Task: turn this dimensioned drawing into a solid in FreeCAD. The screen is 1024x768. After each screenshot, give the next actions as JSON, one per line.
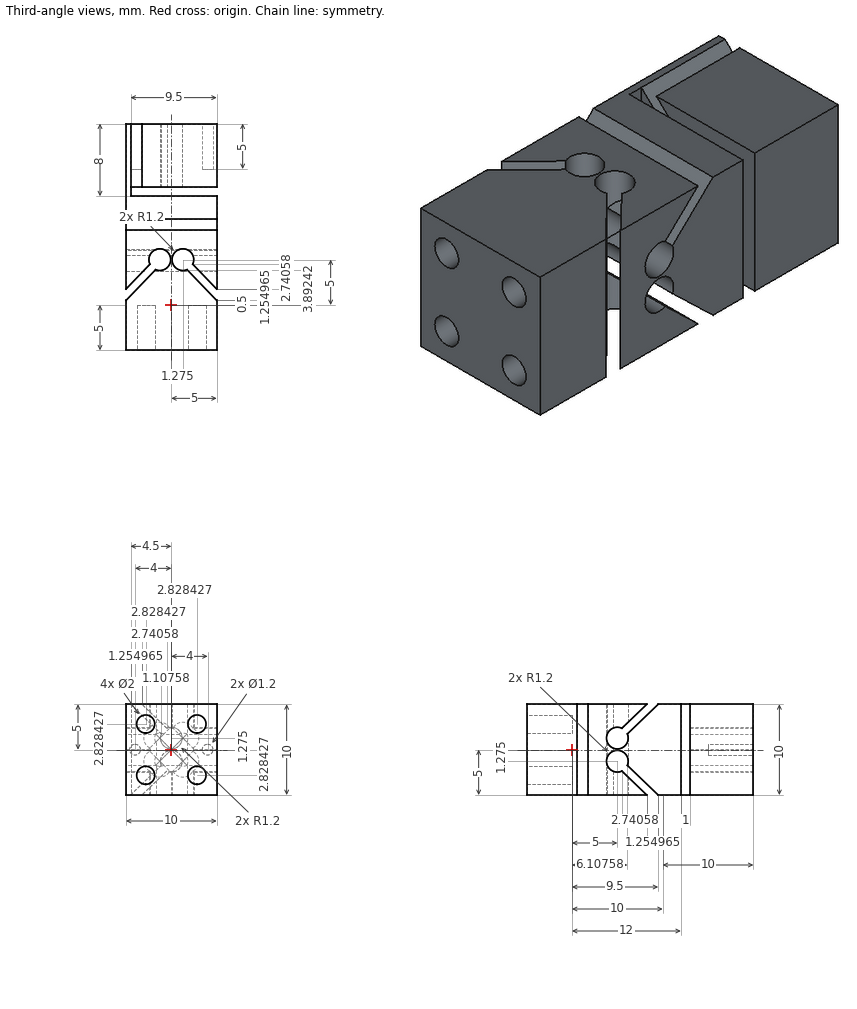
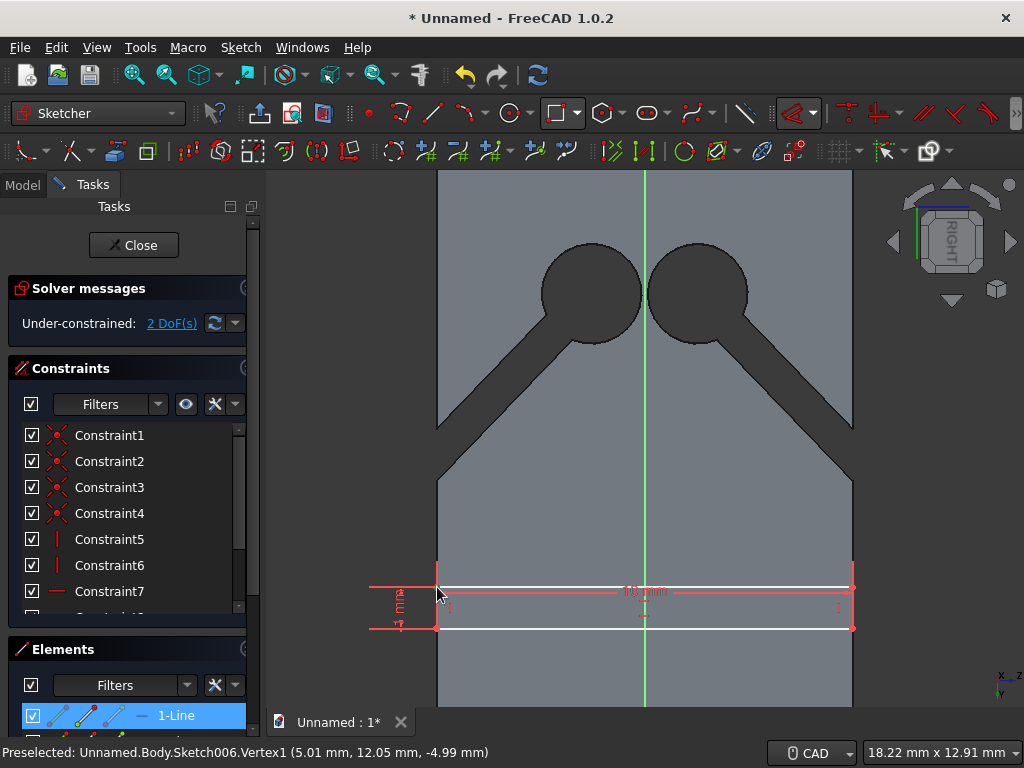
{"action": "key", "text": "l"}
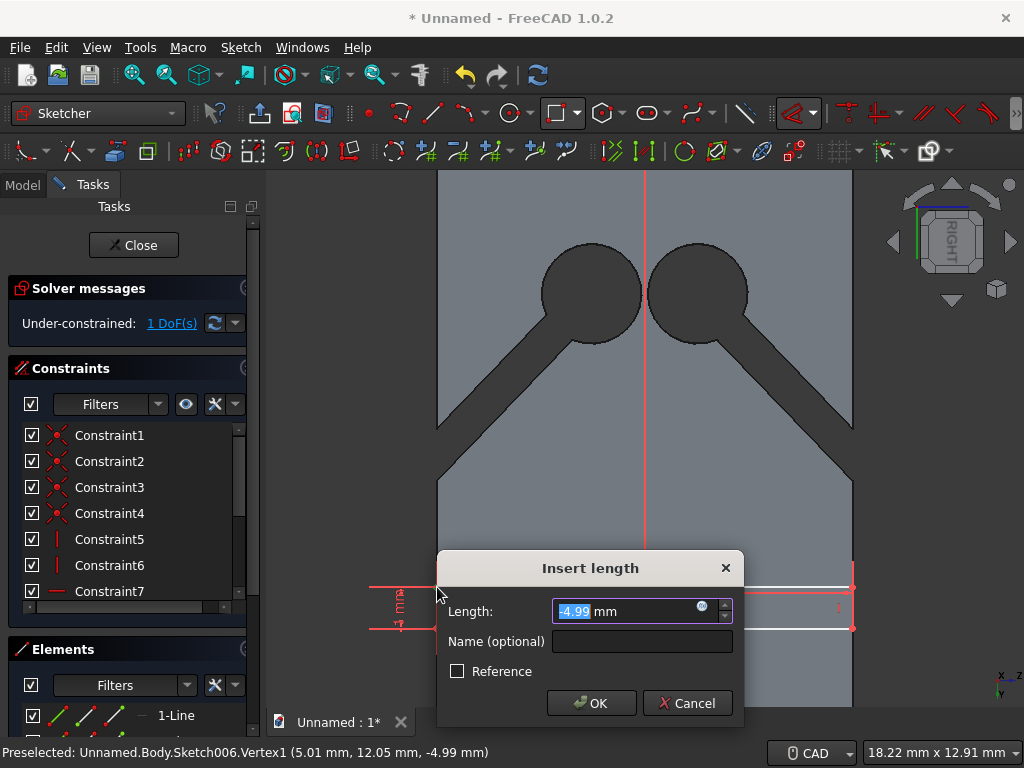
{"action": "type", "text": "-5"}
{"action": "key", "text": "Return"}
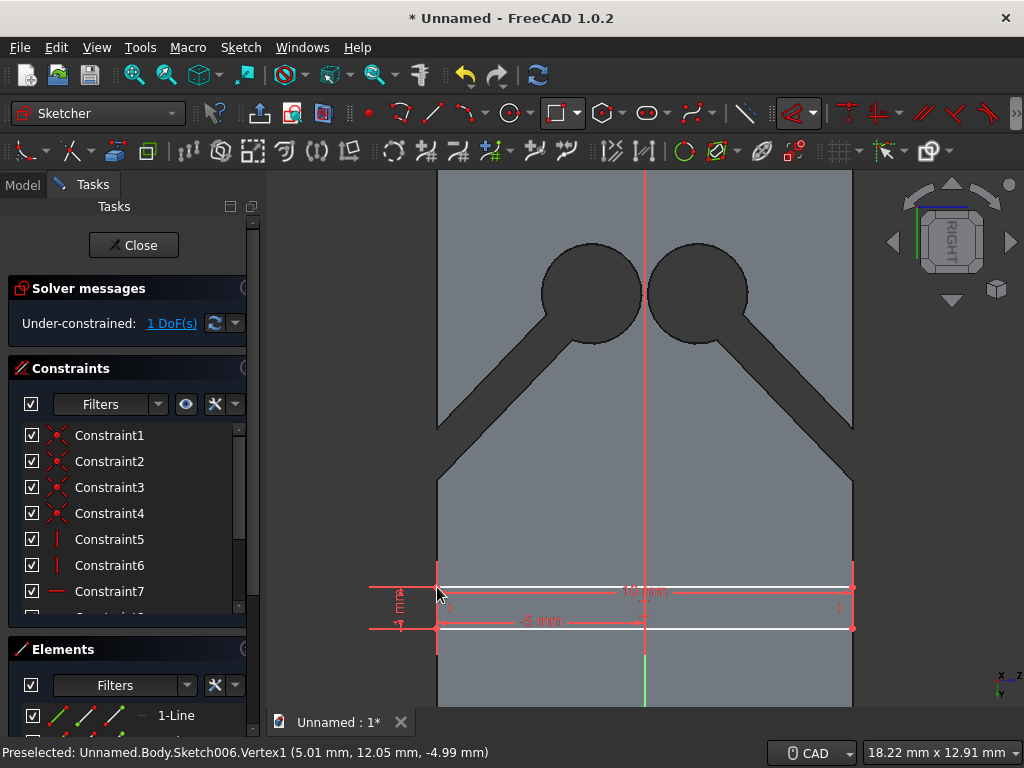
{"action": "left_click", "coordinate": [437, 587]}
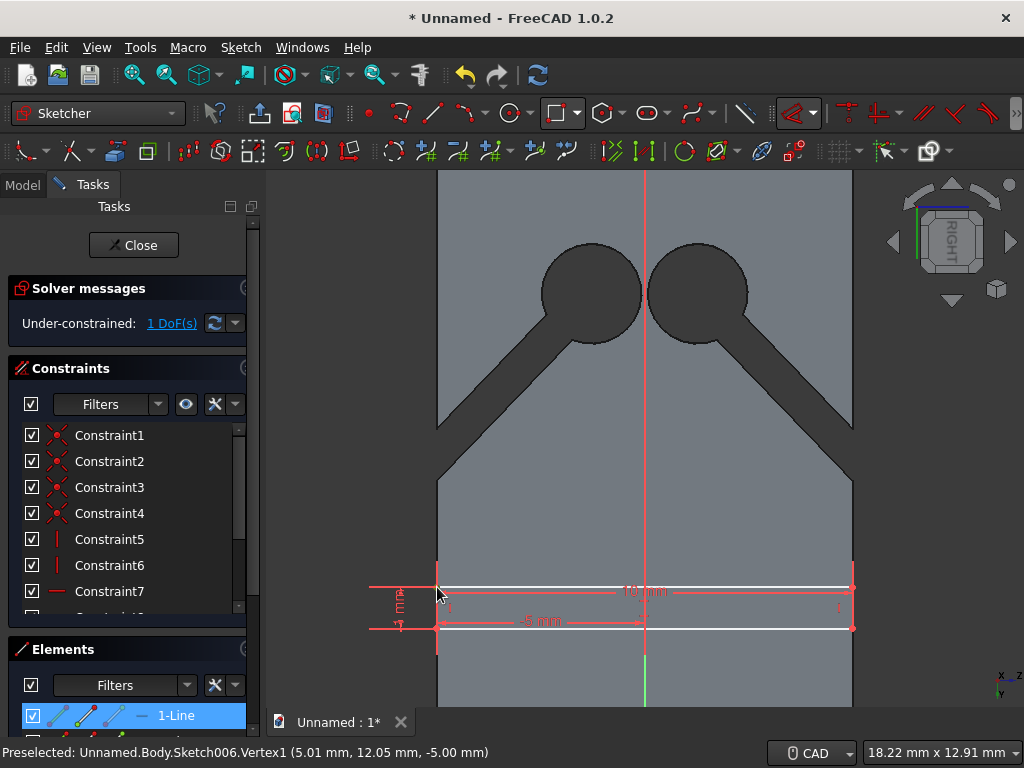
{"action": "key", "text": "i"}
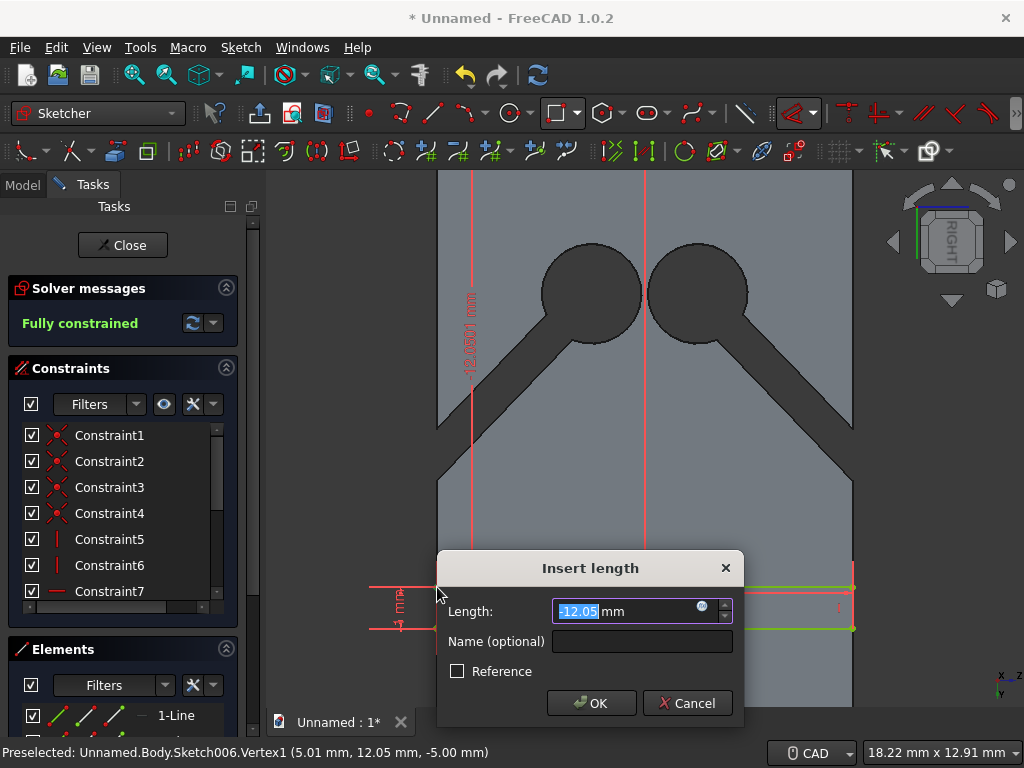
{"action": "type", "text": "-12"}
{"action": "key", "text": "Return"}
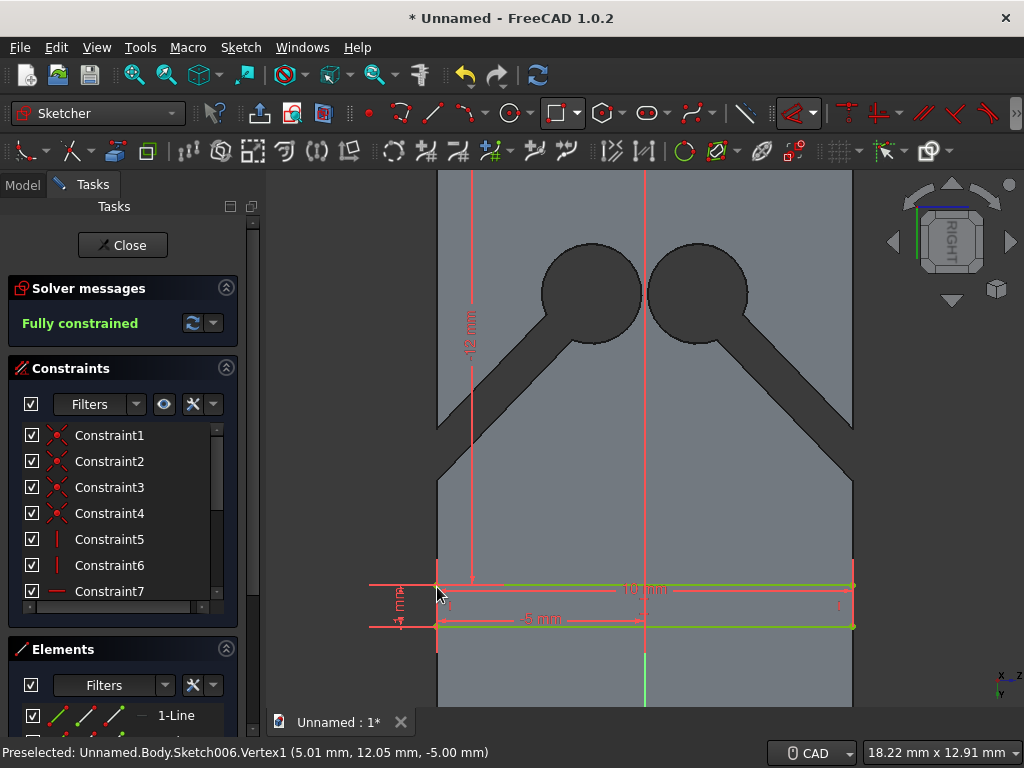
{"action": "left_click", "coordinate": [123, 245]}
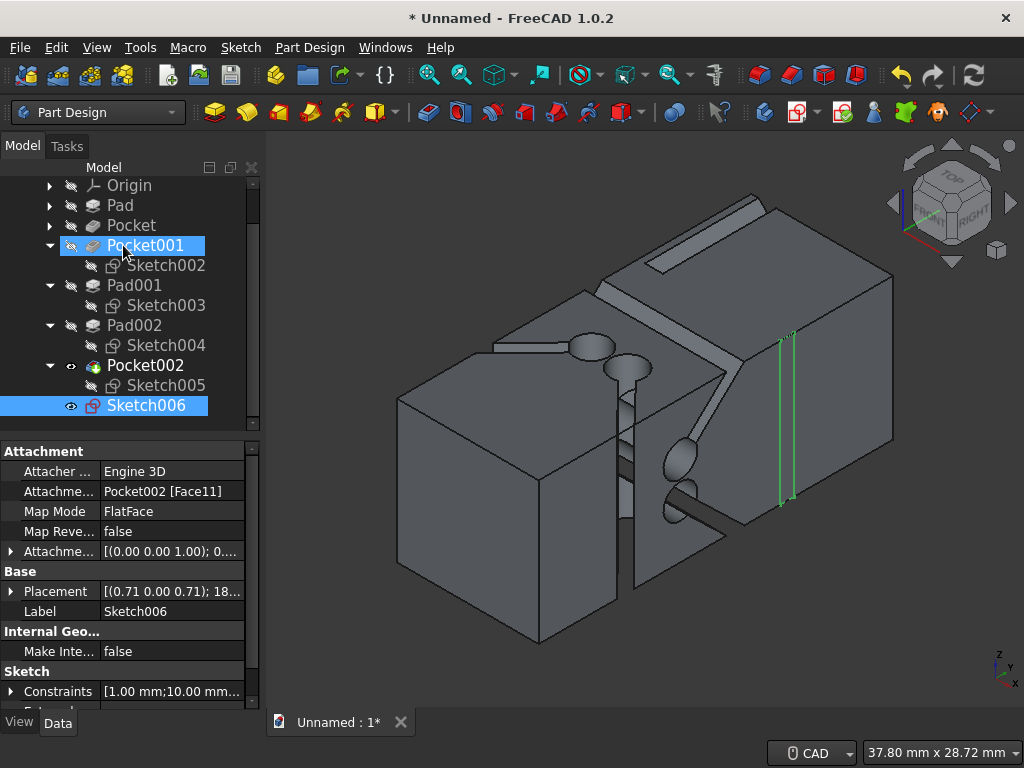
{"action": "left_click", "coordinate": [430, 112]}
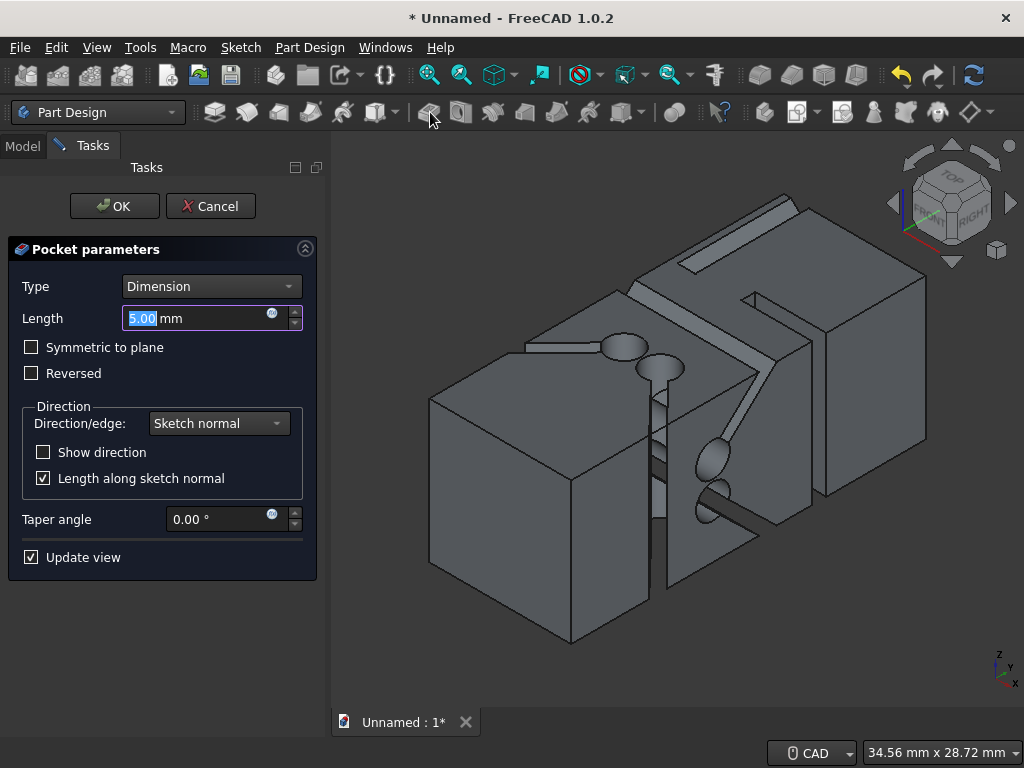
{"action": "type", "text": "9.5"}
{"action": "key", "text": "Tab"}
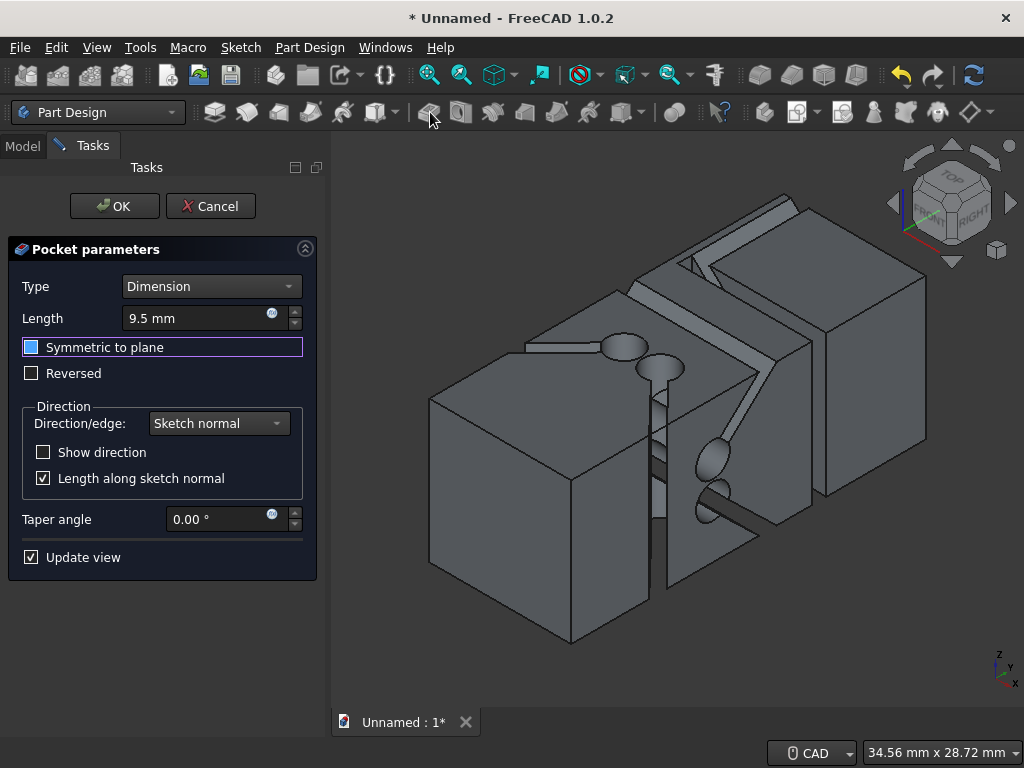
{"action": "left_click", "coordinate": [115, 206]}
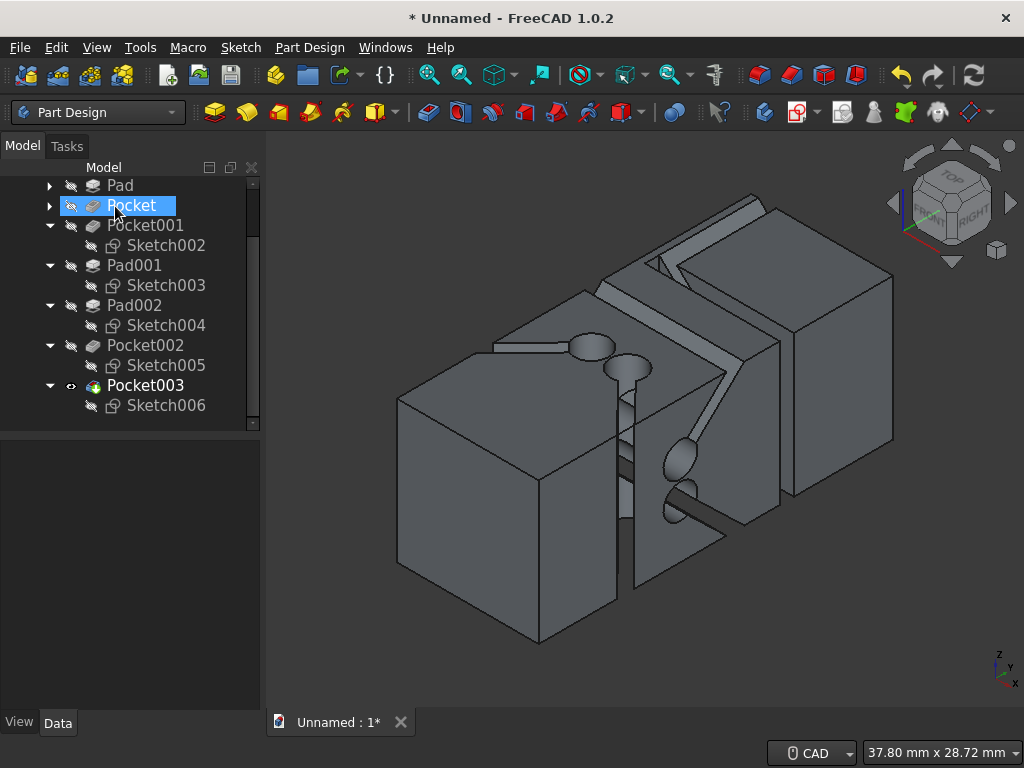
{"action": "left_click", "coordinate": [468, 520]}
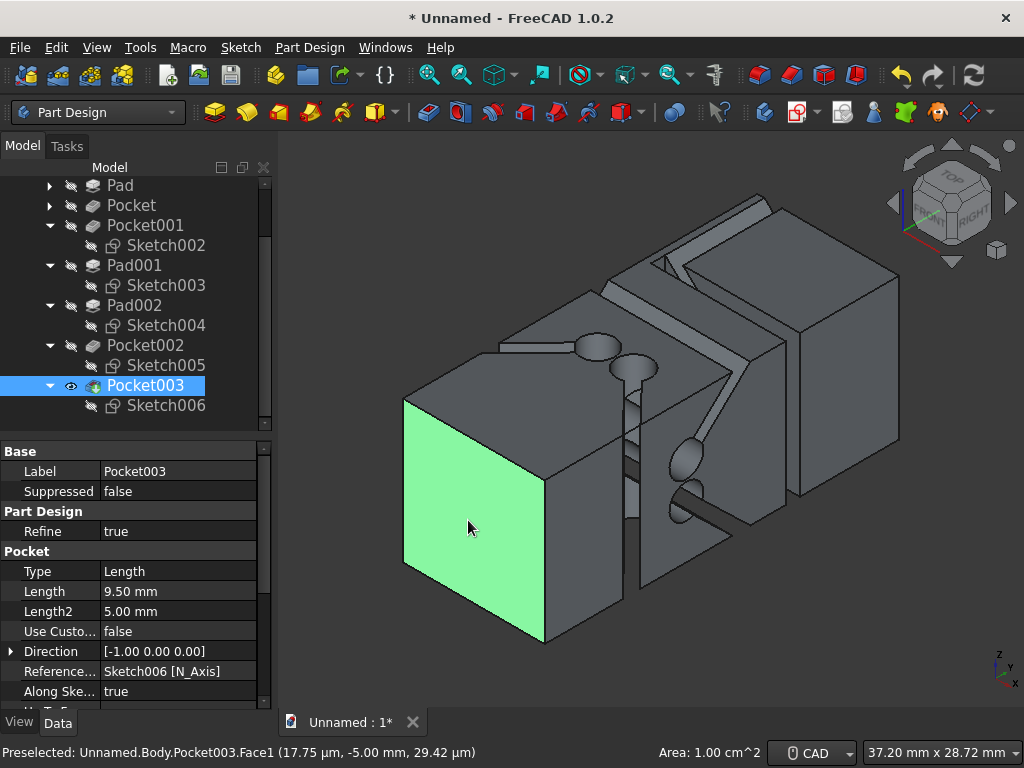
{"action": "left_click", "coordinate": [798, 112]}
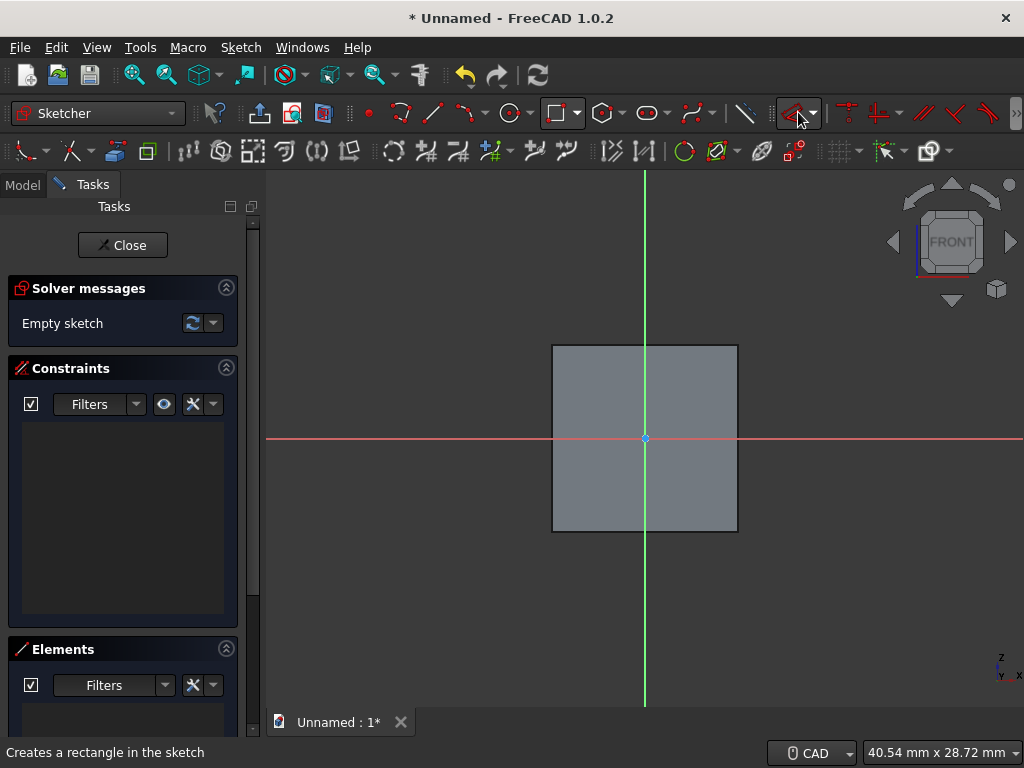
{"action": "scroll", "coordinate": [701, 439], "scroll_direction": "up", "scroll_amount": 4}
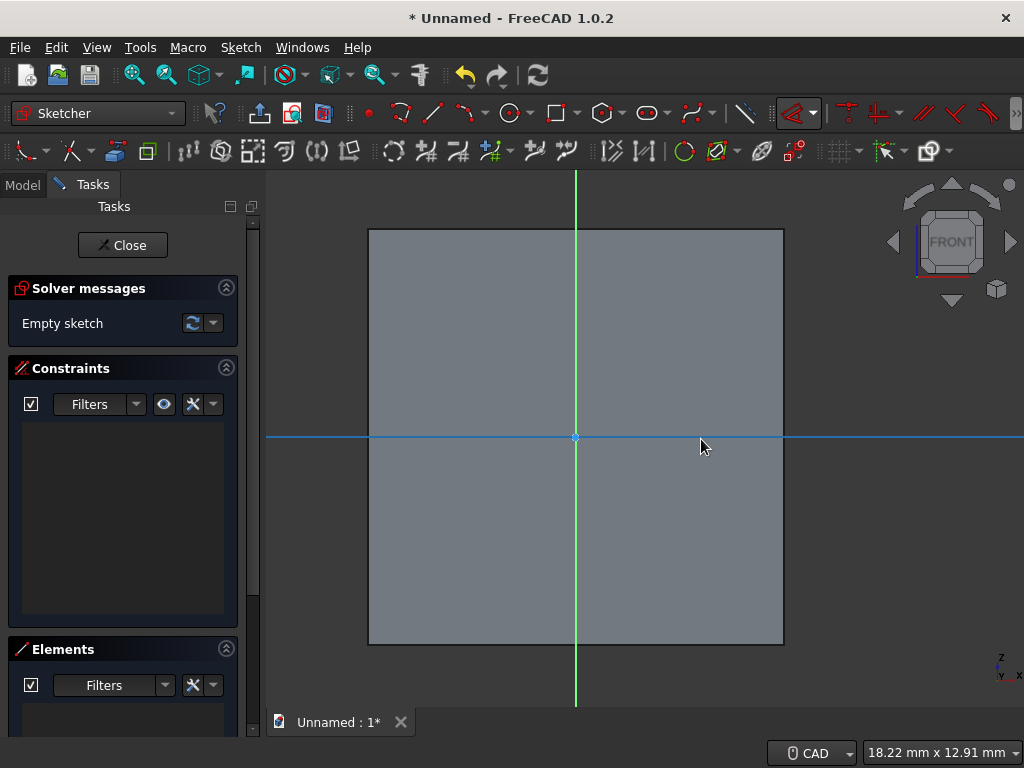
{"action": "left_click", "coordinate": [510, 114]}